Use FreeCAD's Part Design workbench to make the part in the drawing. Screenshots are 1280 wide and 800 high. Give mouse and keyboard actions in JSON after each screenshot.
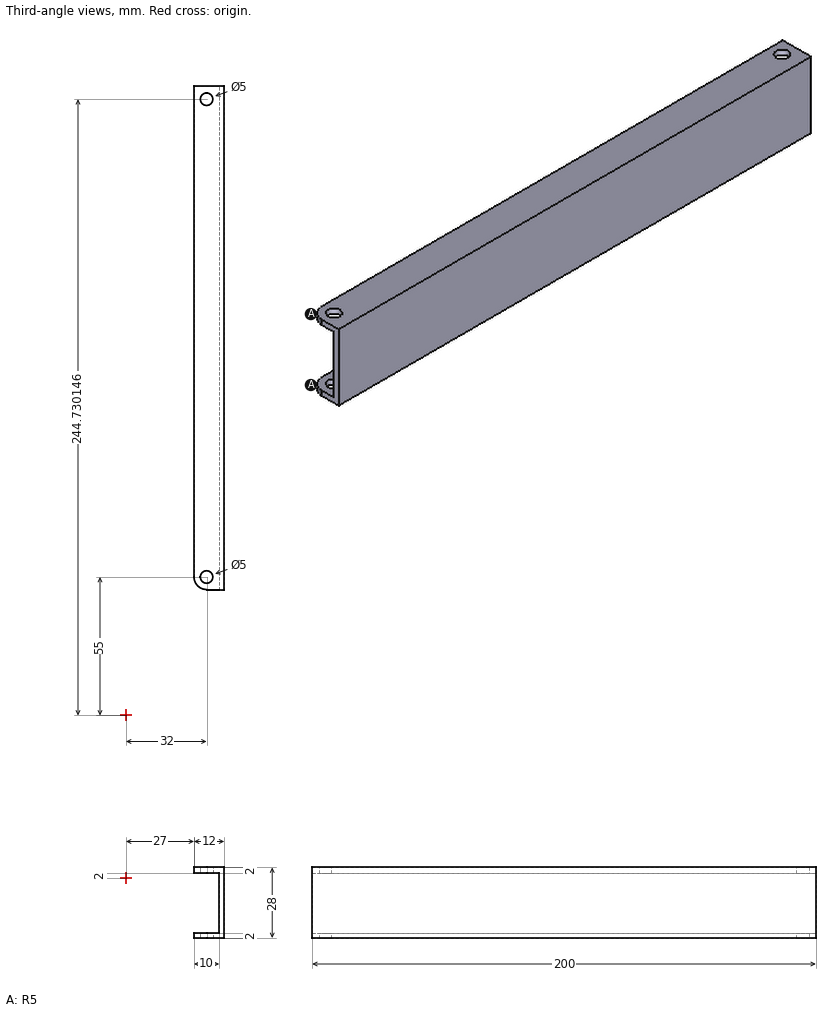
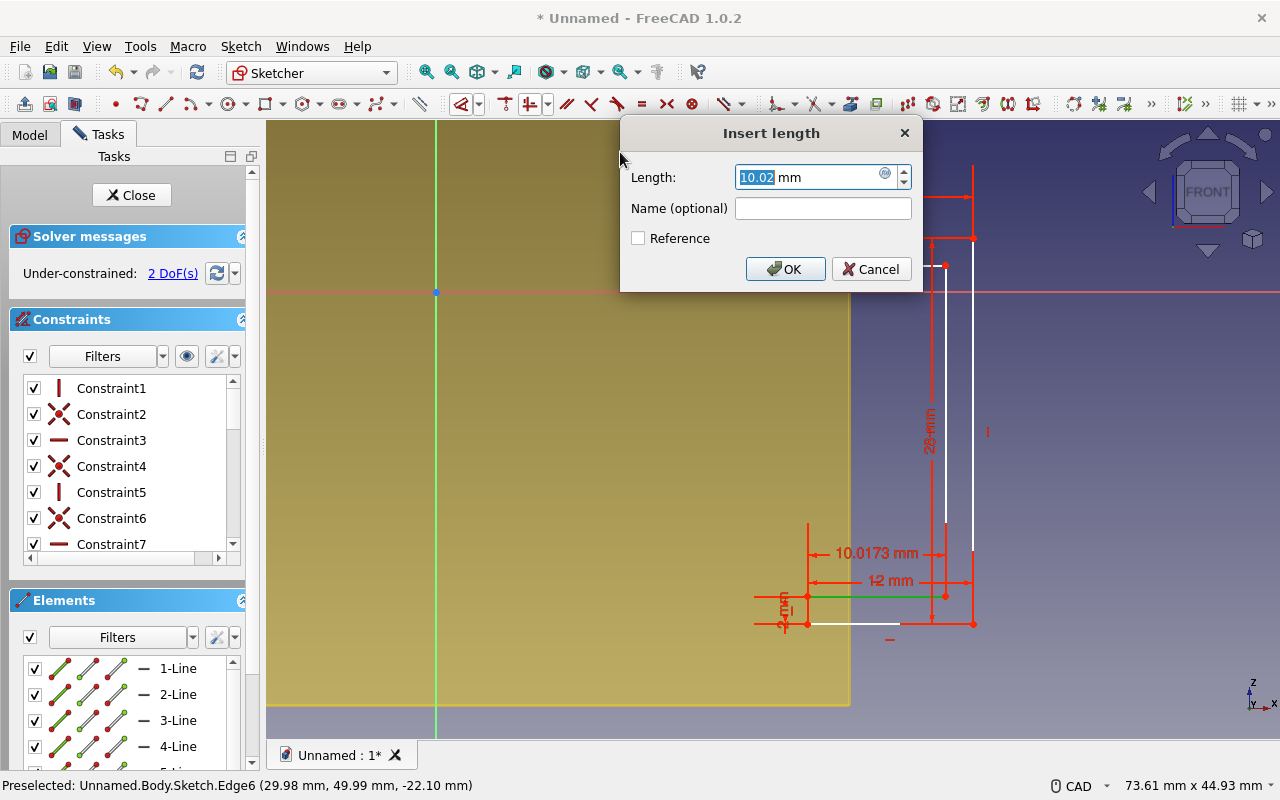
{"action": "type", "text": "10"}
{"action": "key", "text": "Return"}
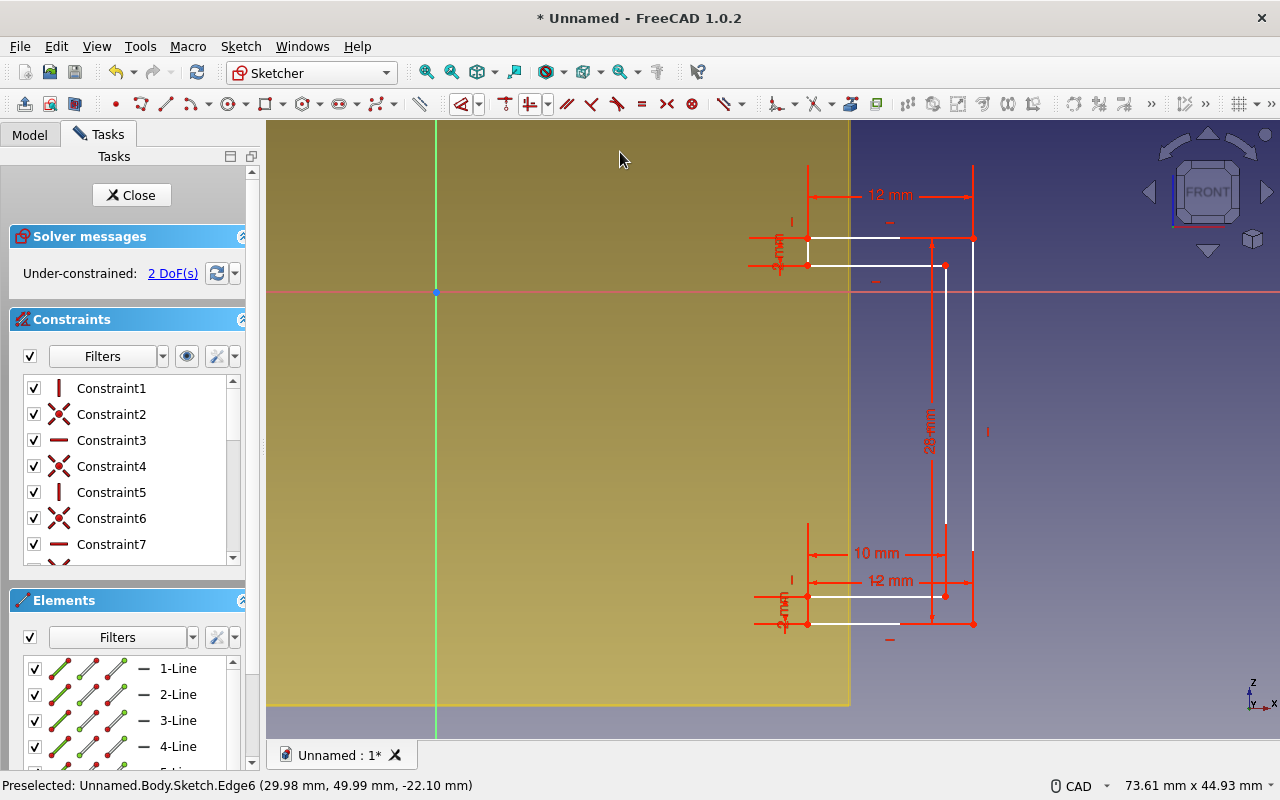
{"action": "scroll", "coordinate": [808, 266], "scroll_direction": "up", "scroll_amount": 2}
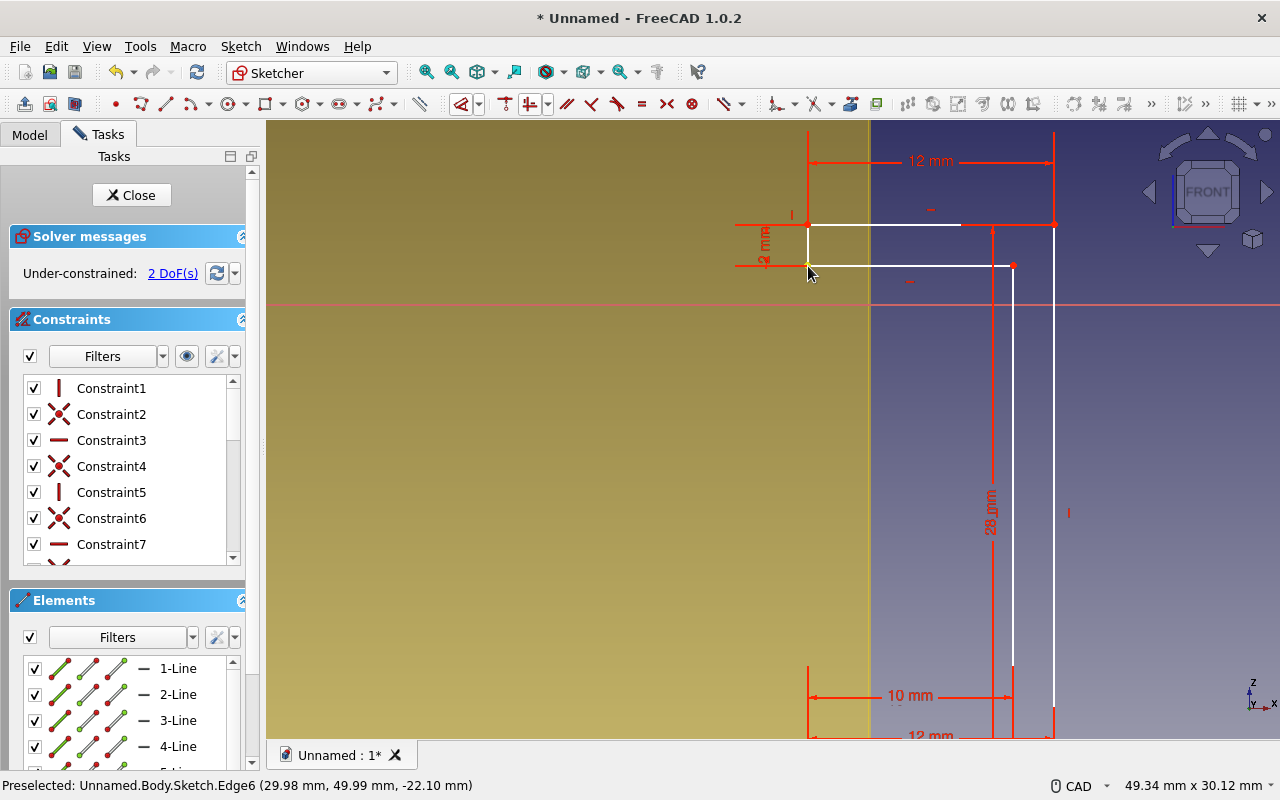
{"action": "left_click", "coordinate": [808, 266]}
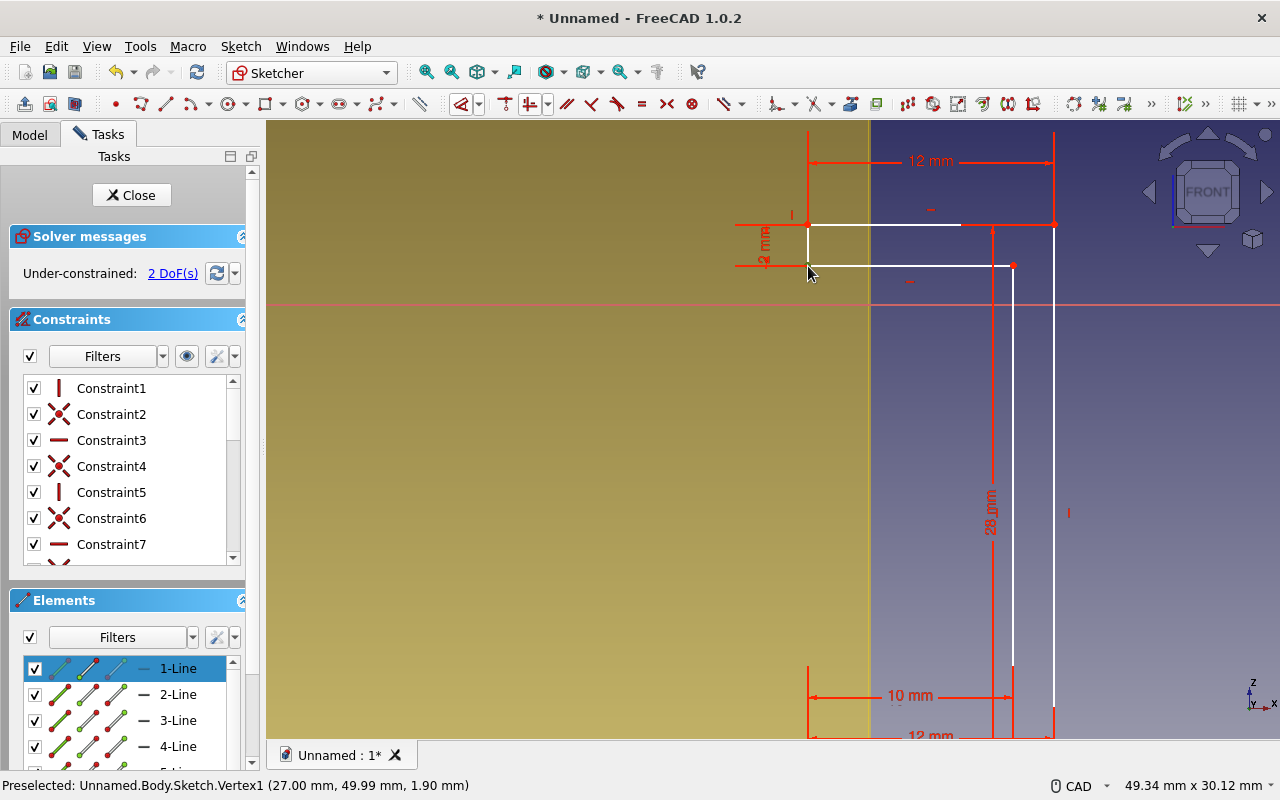
{"action": "left_click", "coordinate": [478, 104]}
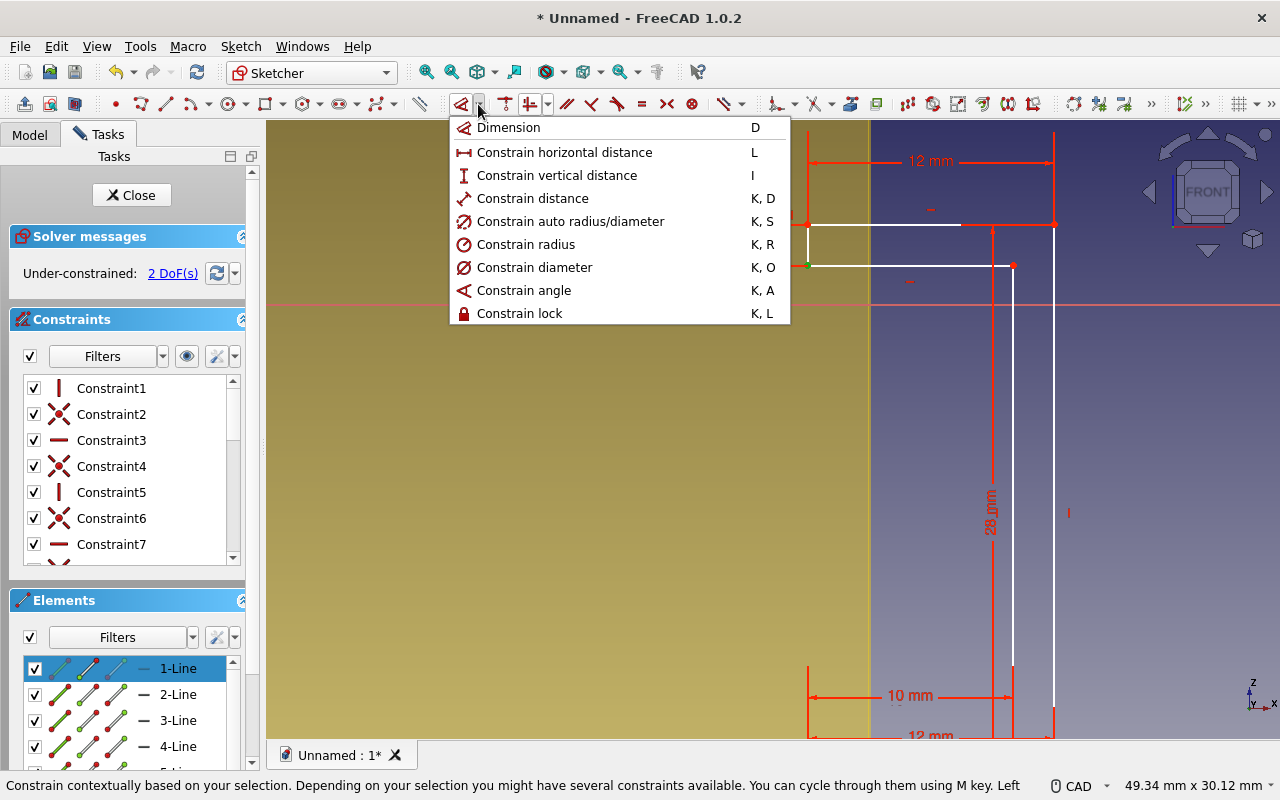
{"action": "left_click", "coordinate": [620, 176]}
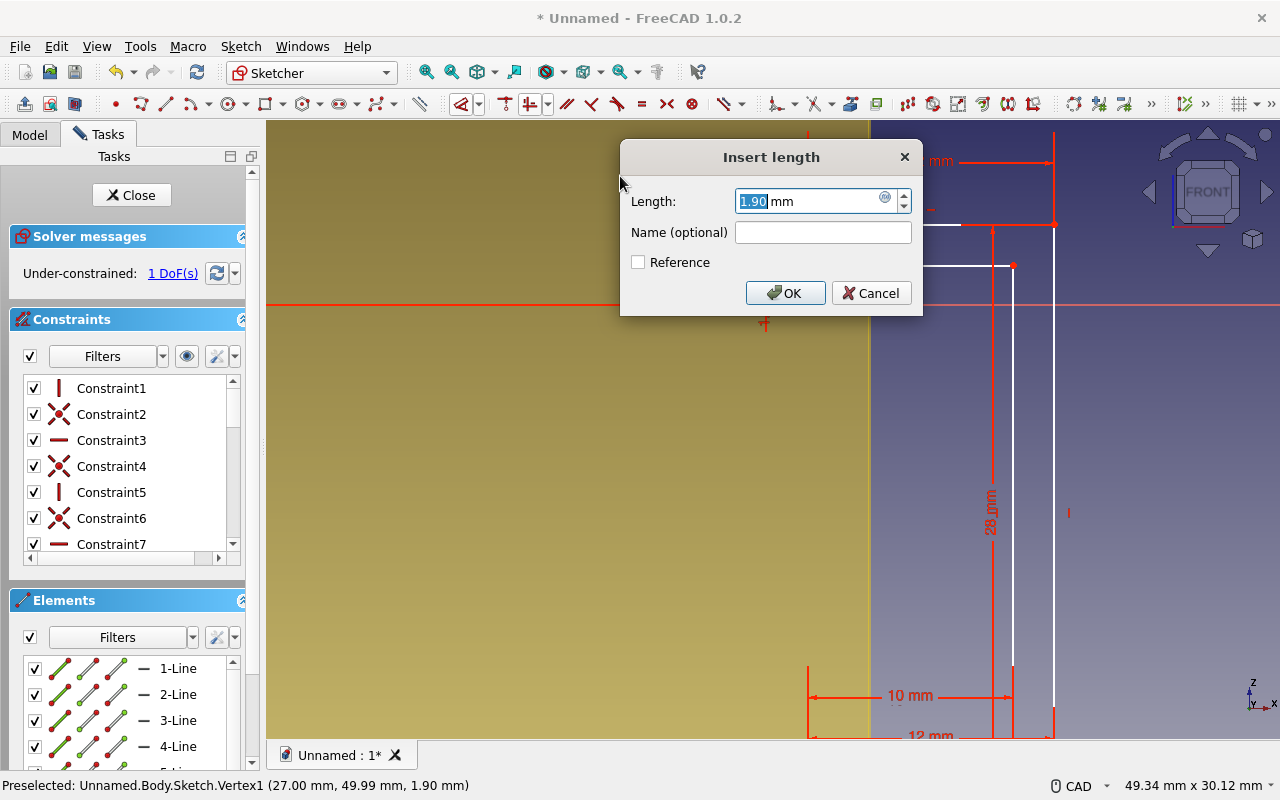
{"action": "type", "text": "2"}
{"action": "key", "text": "Return"}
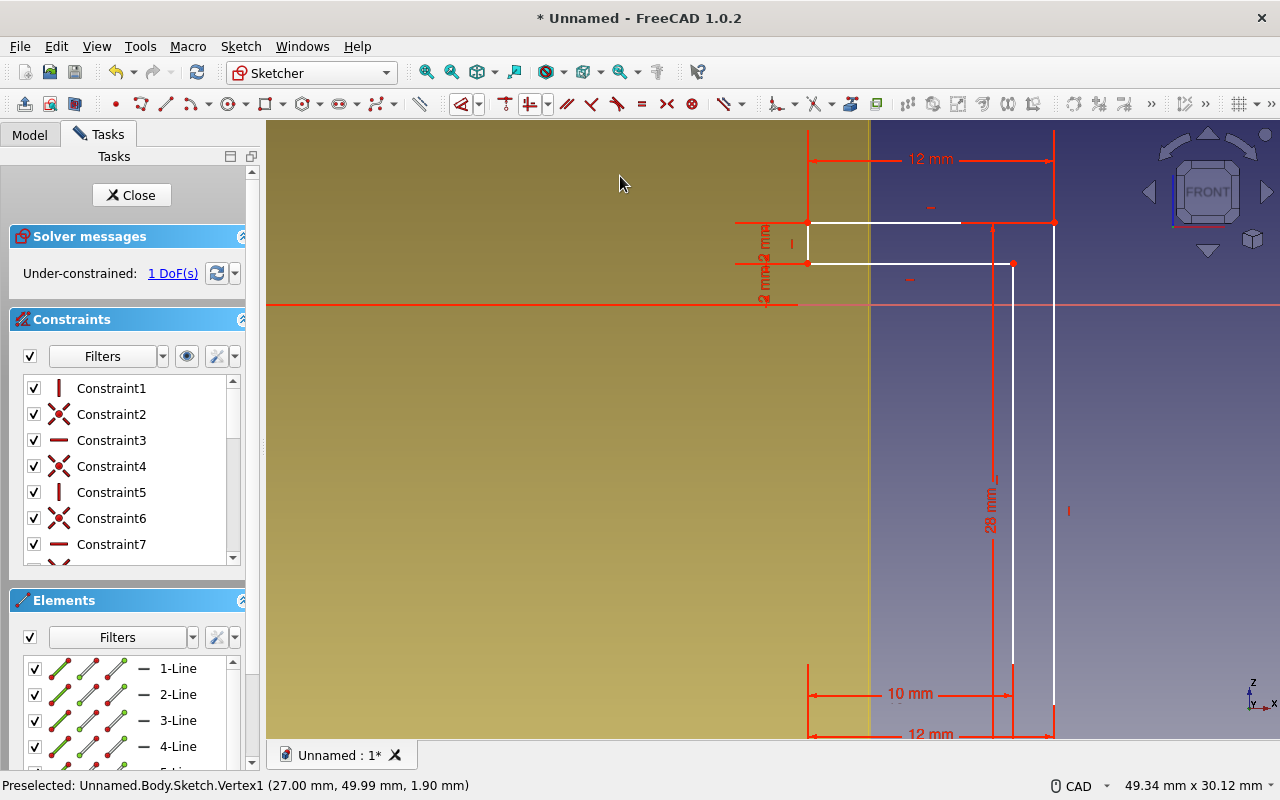
{"action": "left_click", "coordinate": [808, 264]}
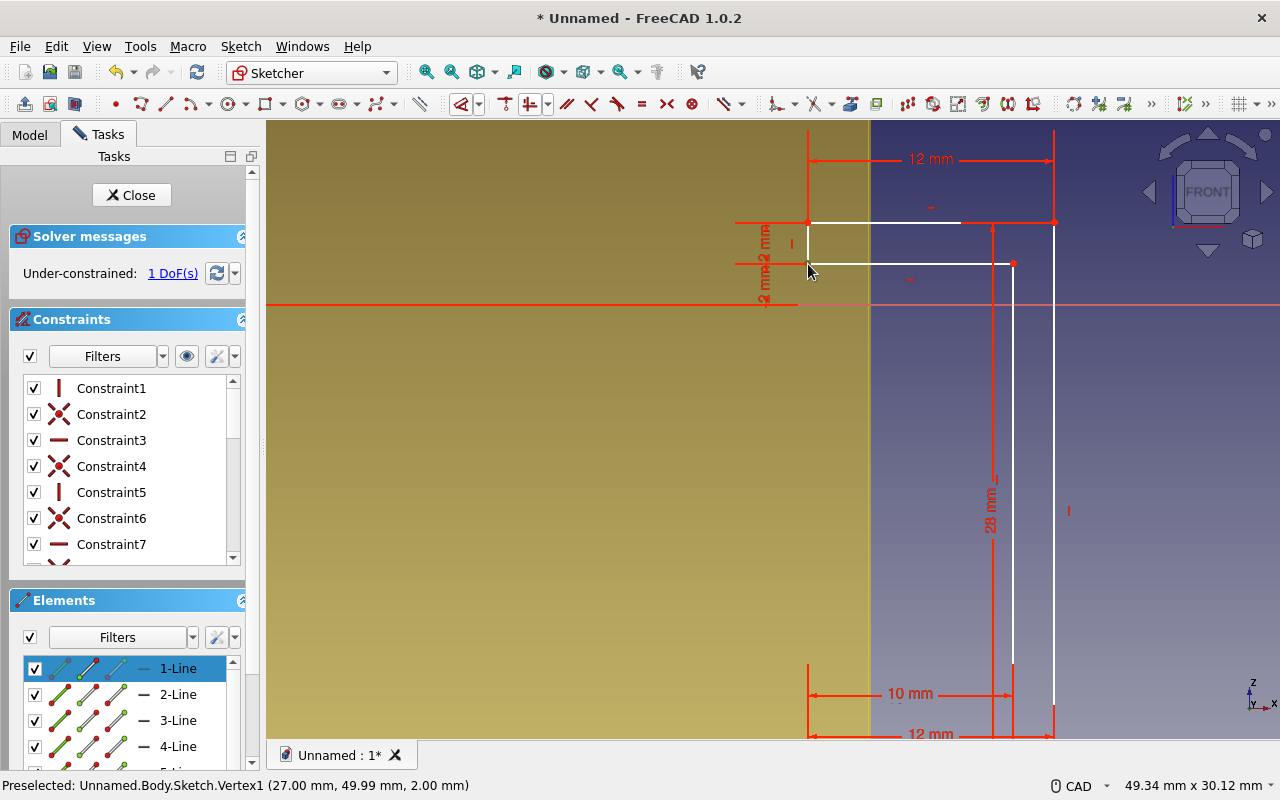
{"action": "left_click", "coordinate": [478, 104]}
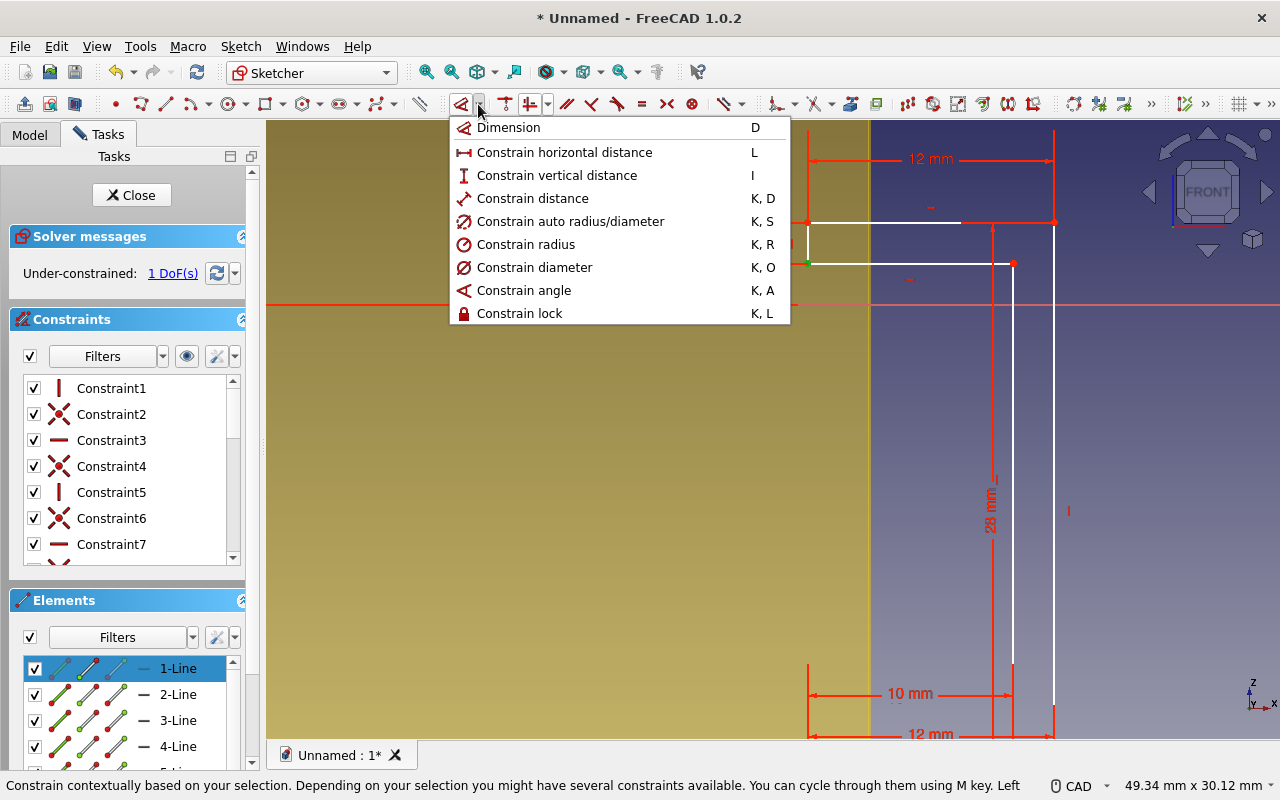
{"action": "left_click", "coordinate": [620, 152]}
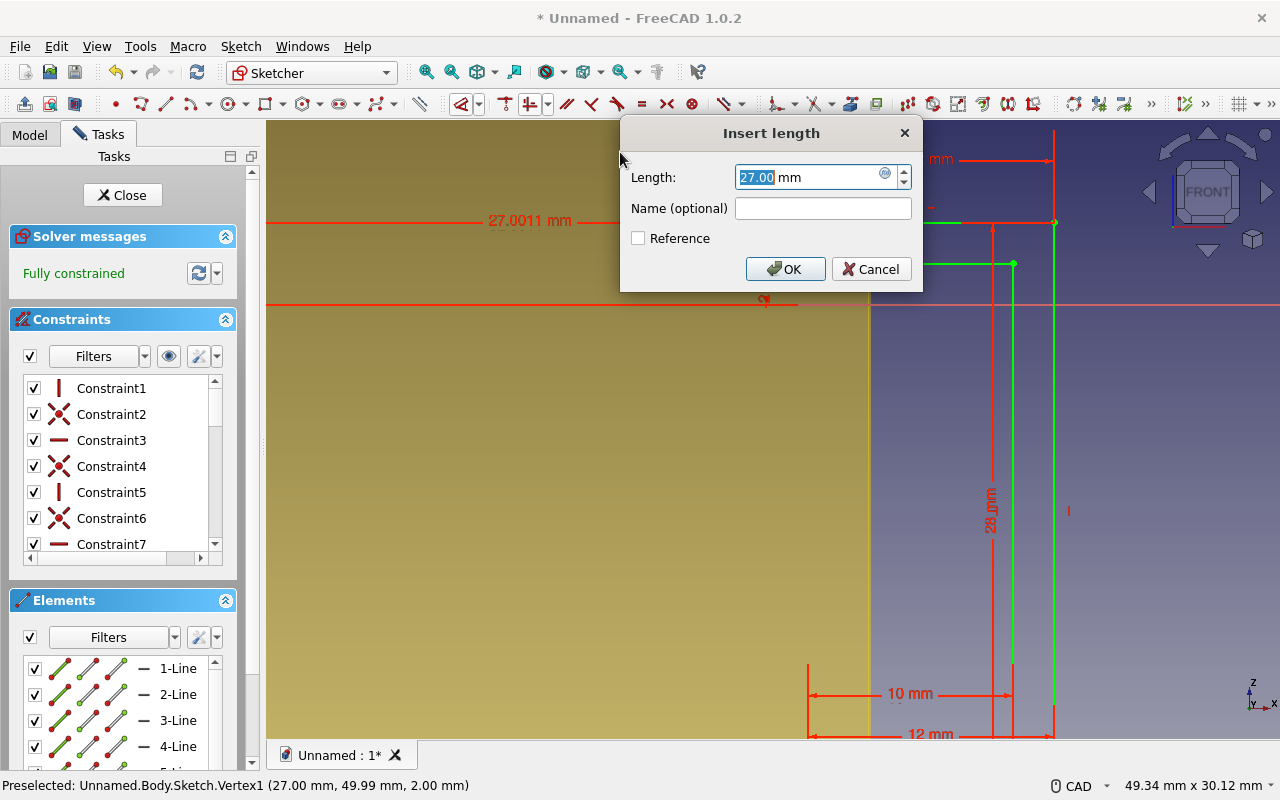
{"action": "type", "text": "27"}
{"action": "key", "text": "Return"}